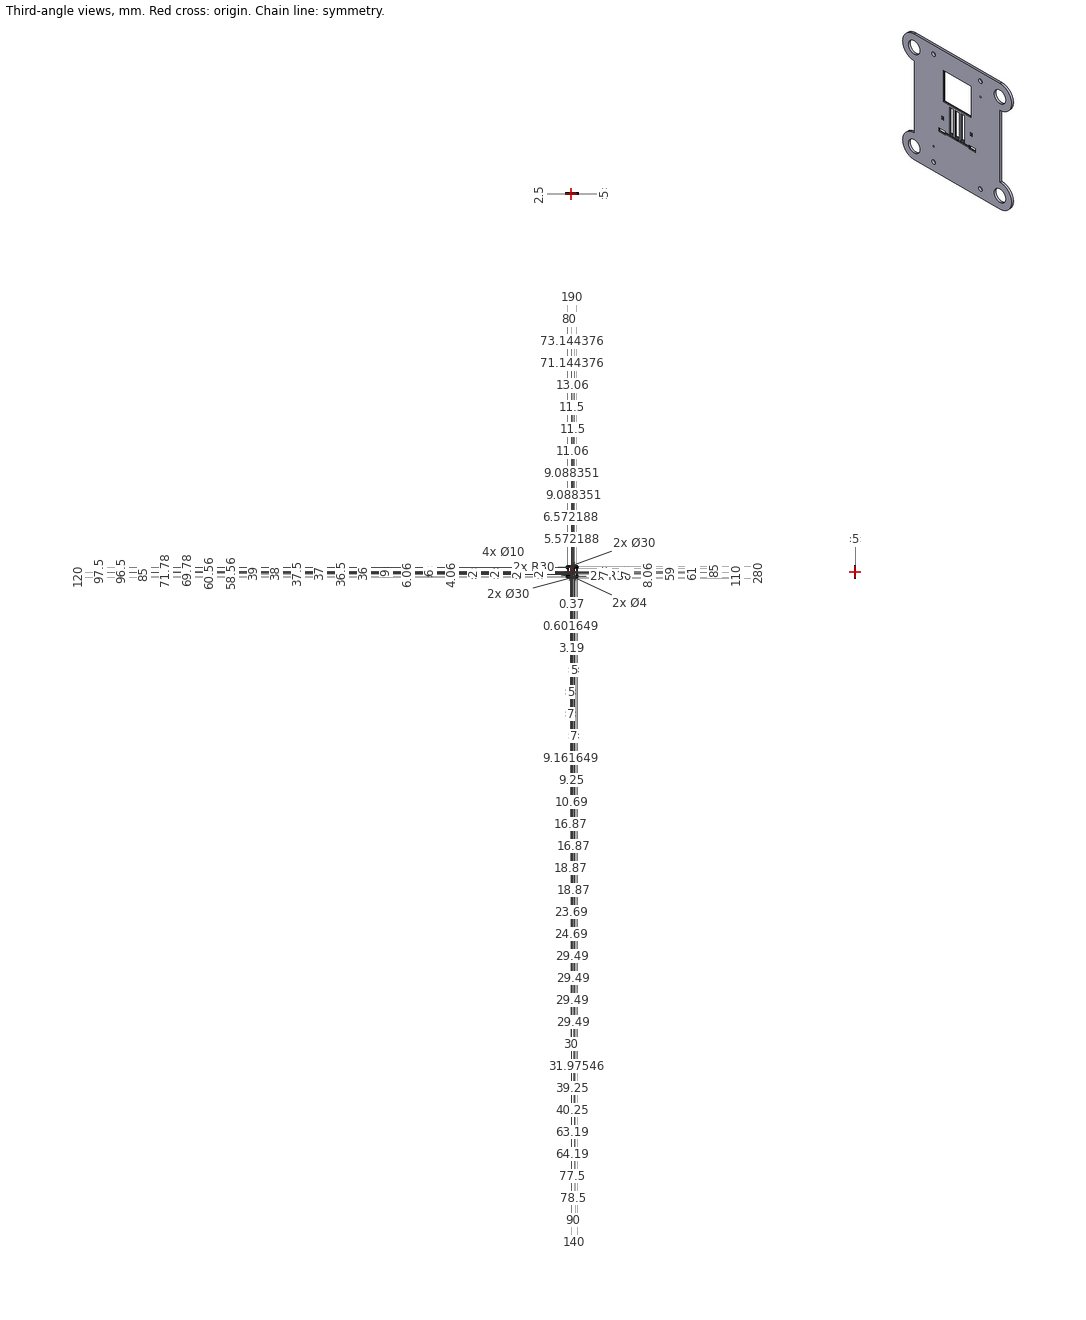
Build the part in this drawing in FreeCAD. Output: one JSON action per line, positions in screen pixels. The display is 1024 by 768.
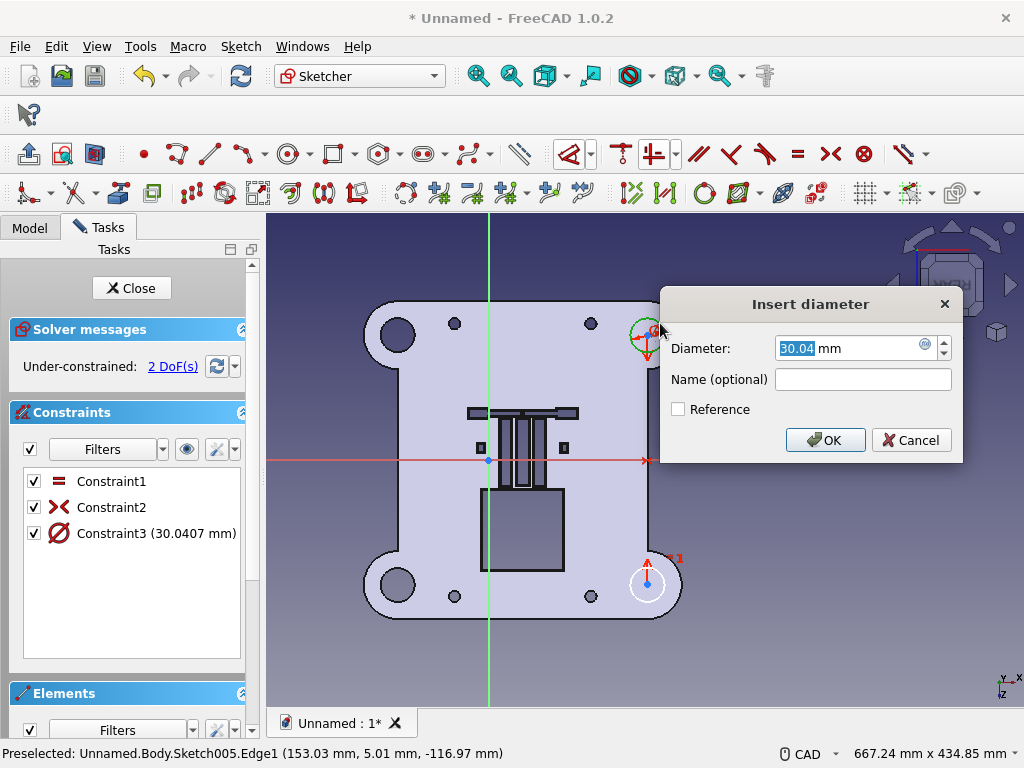
{"action": "type", "text": "30"}
{"action": "key", "text": "Return"}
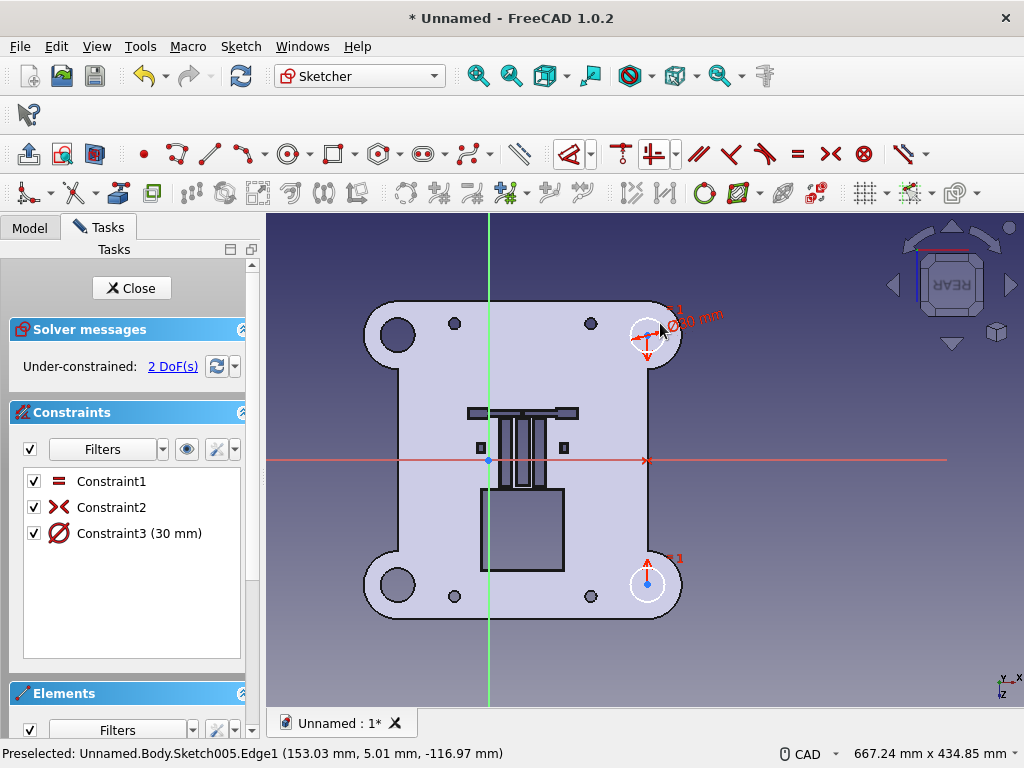
{"action": "left_click", "coordinate": [647, 335]}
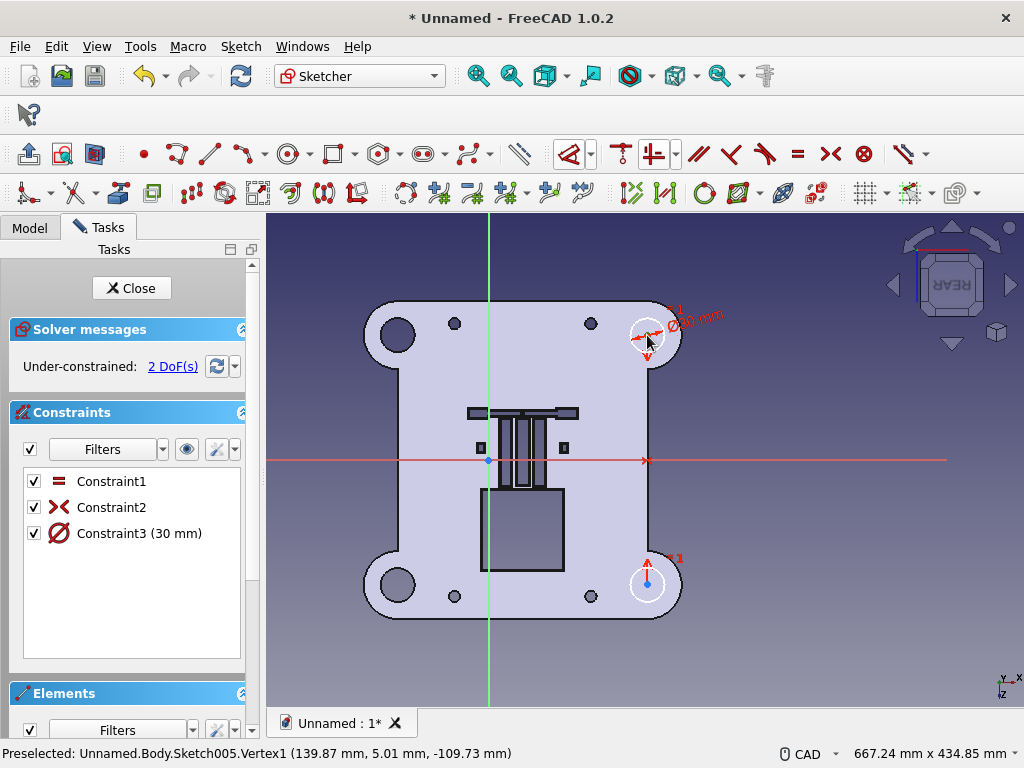
{"action": "key", "text": "l"}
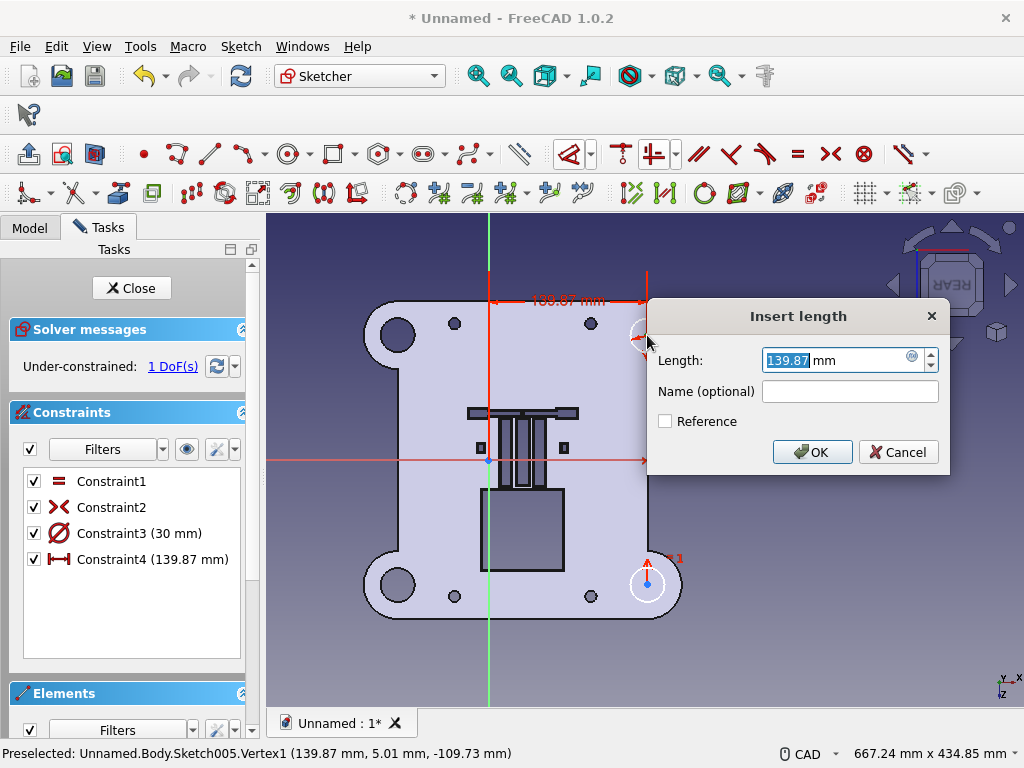
{"action": "type", "text": "140"}
{"action": "key", "text": "Return"}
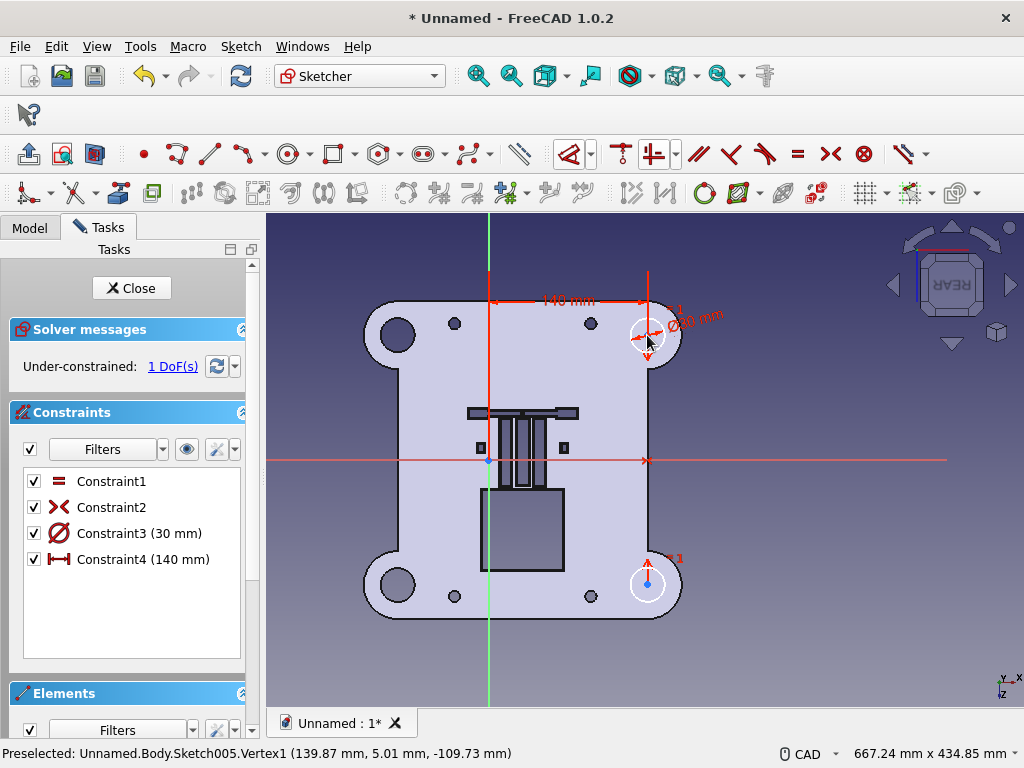
{"action": "left_click", "coordinate": [648, 335]}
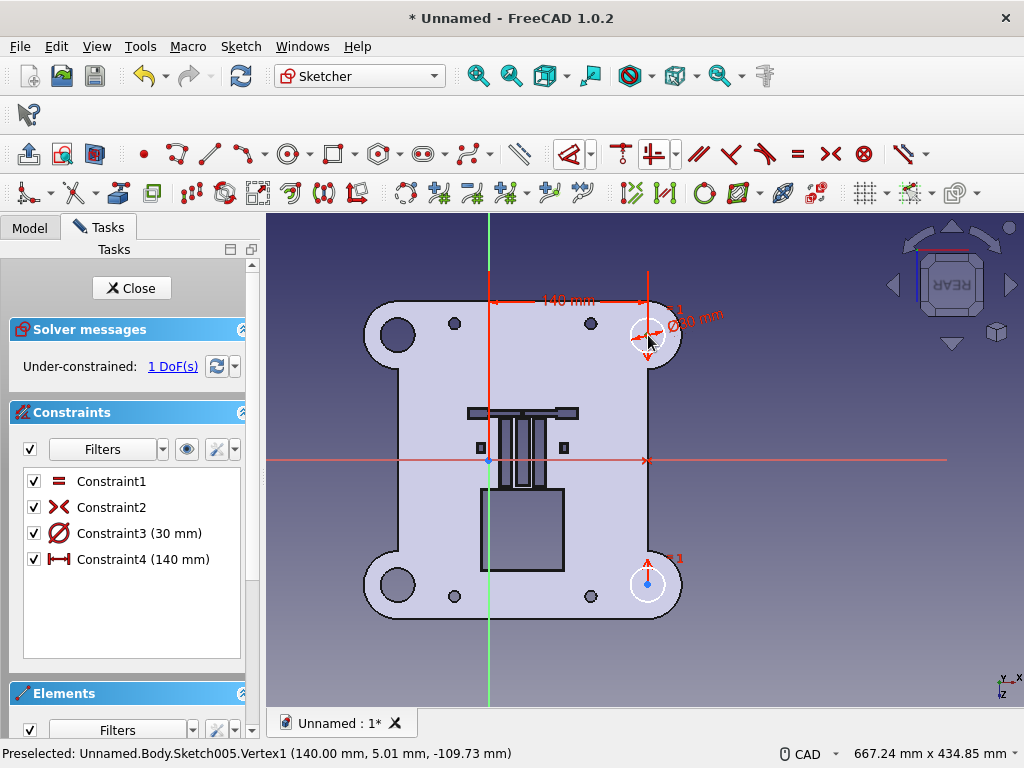
{"action": "key", "text": "i"}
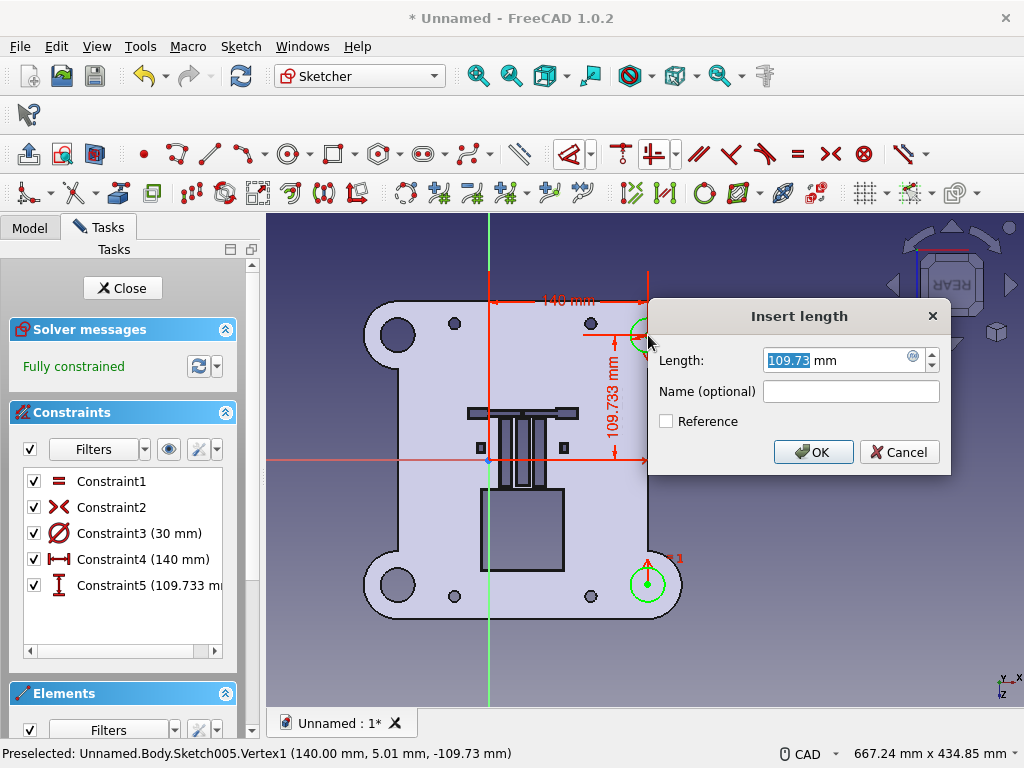
{"action": "type", "text": "110"}
{"action": "key", "text": "Return"}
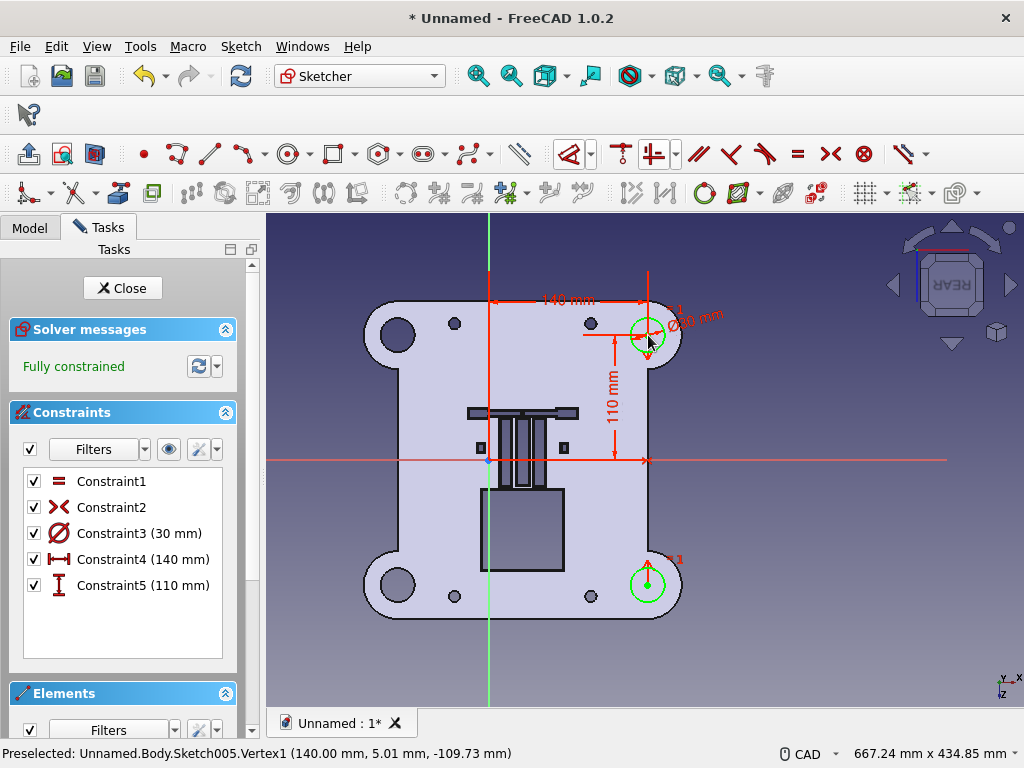
{"action": "left_click", "coordinate": [123, 288]}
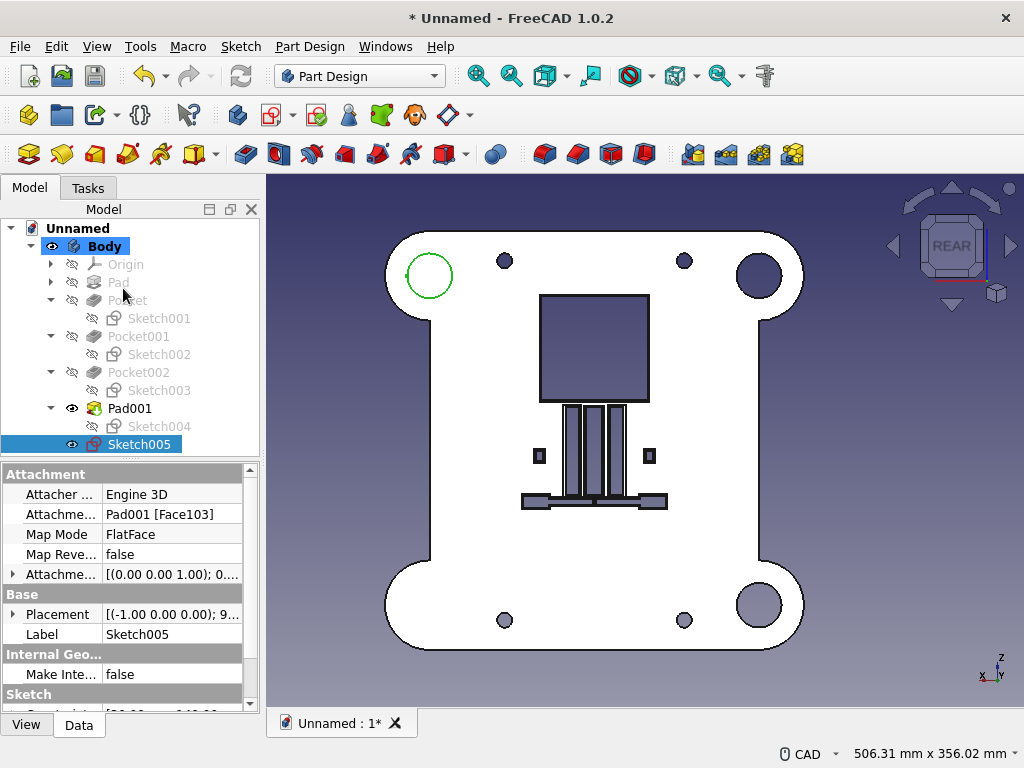
{"action": "left_click", "coordinate": [246, 154]}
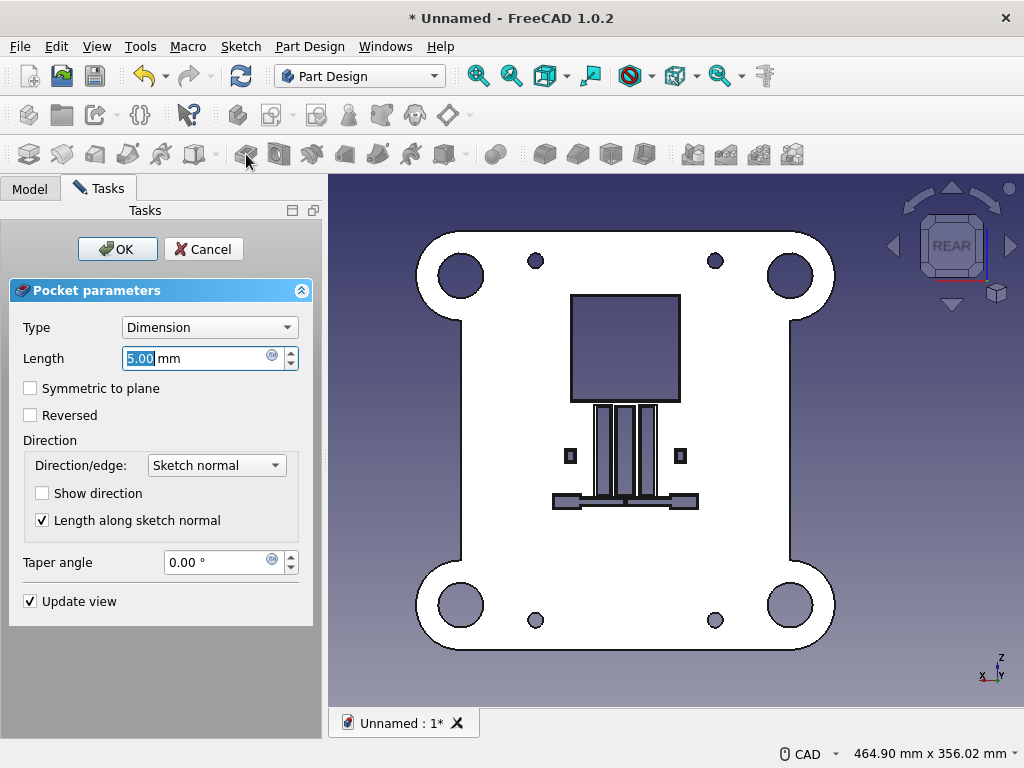
{"action": "type", "text": "5"}
{"action": "key", "text": "Tab"}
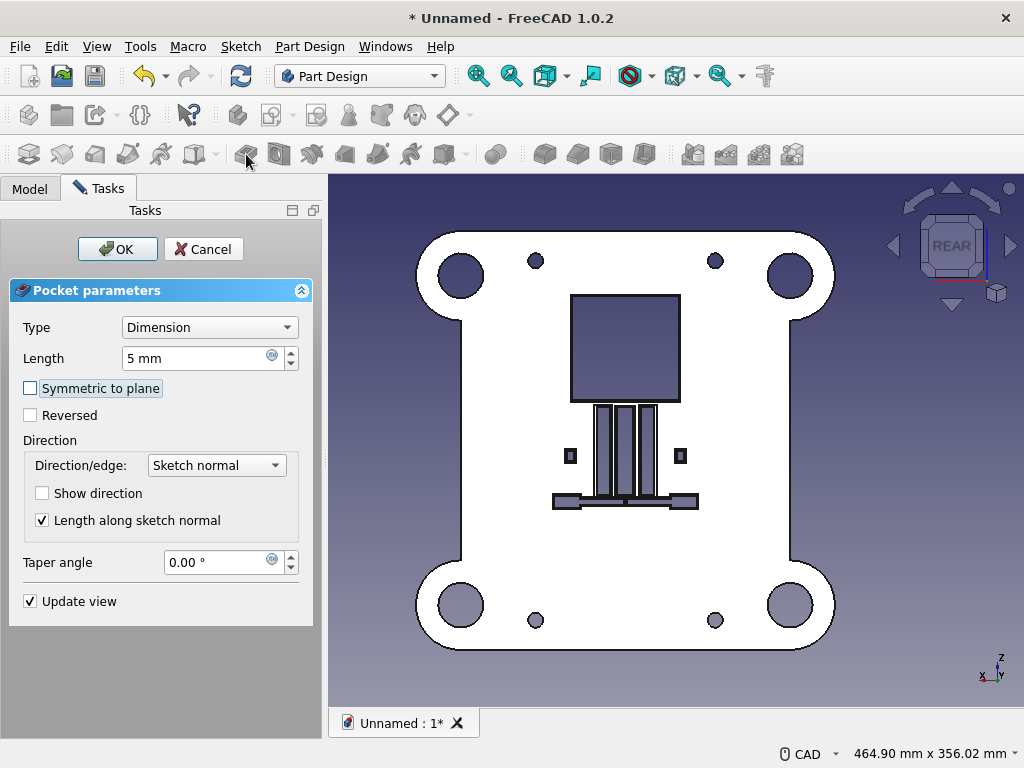
{"action": "left_click", "coordinate": [118, 249]}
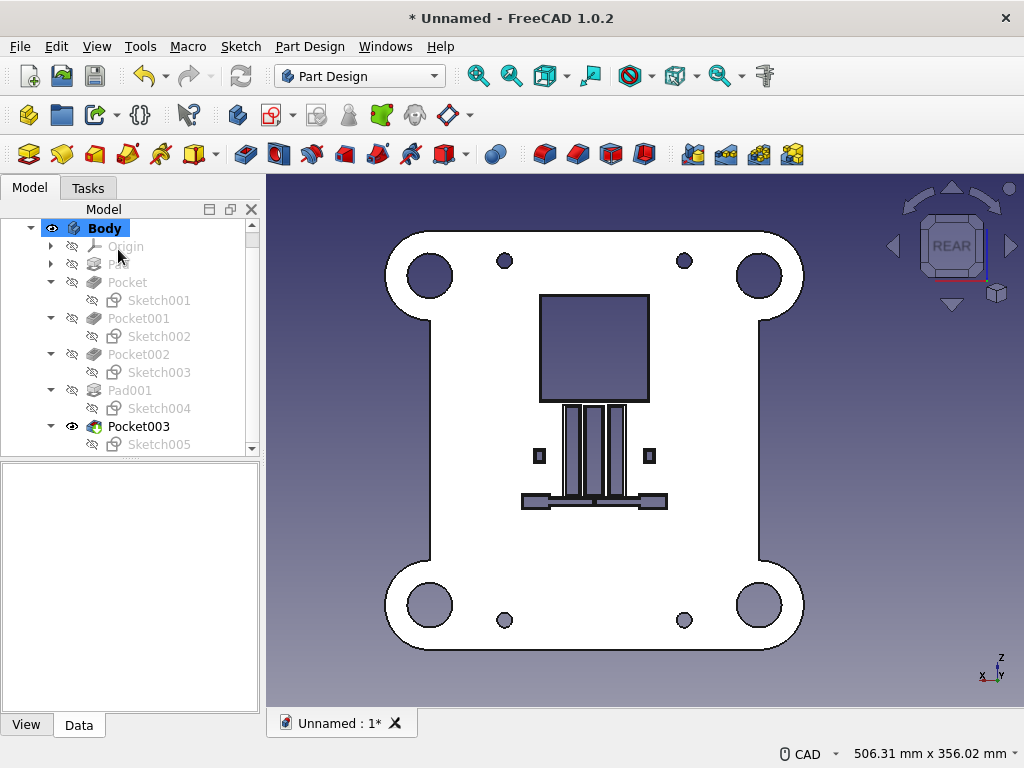
{"action": "left_click", "coordinate": [594, 559]}